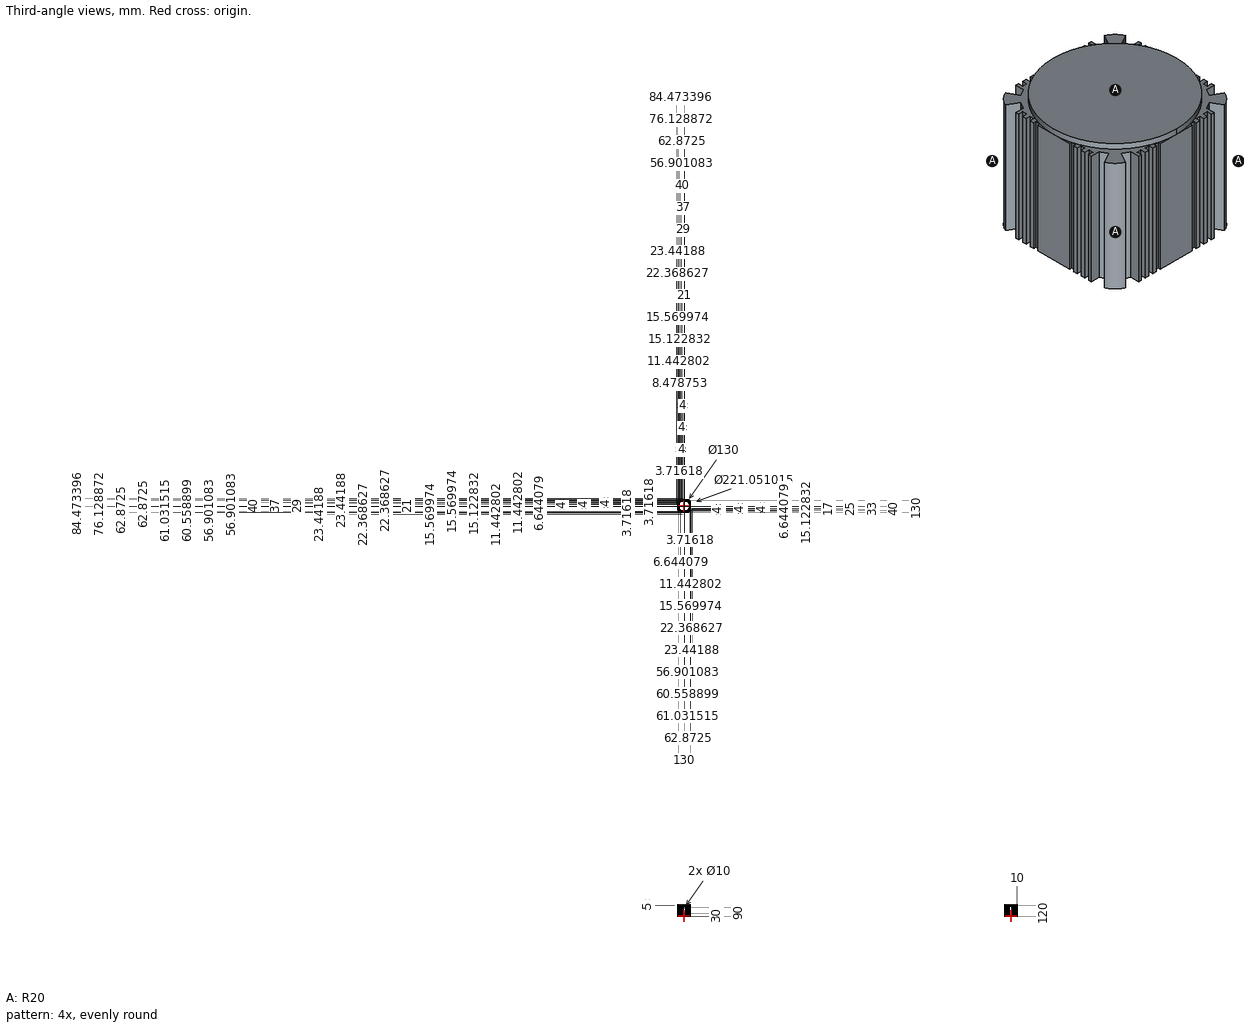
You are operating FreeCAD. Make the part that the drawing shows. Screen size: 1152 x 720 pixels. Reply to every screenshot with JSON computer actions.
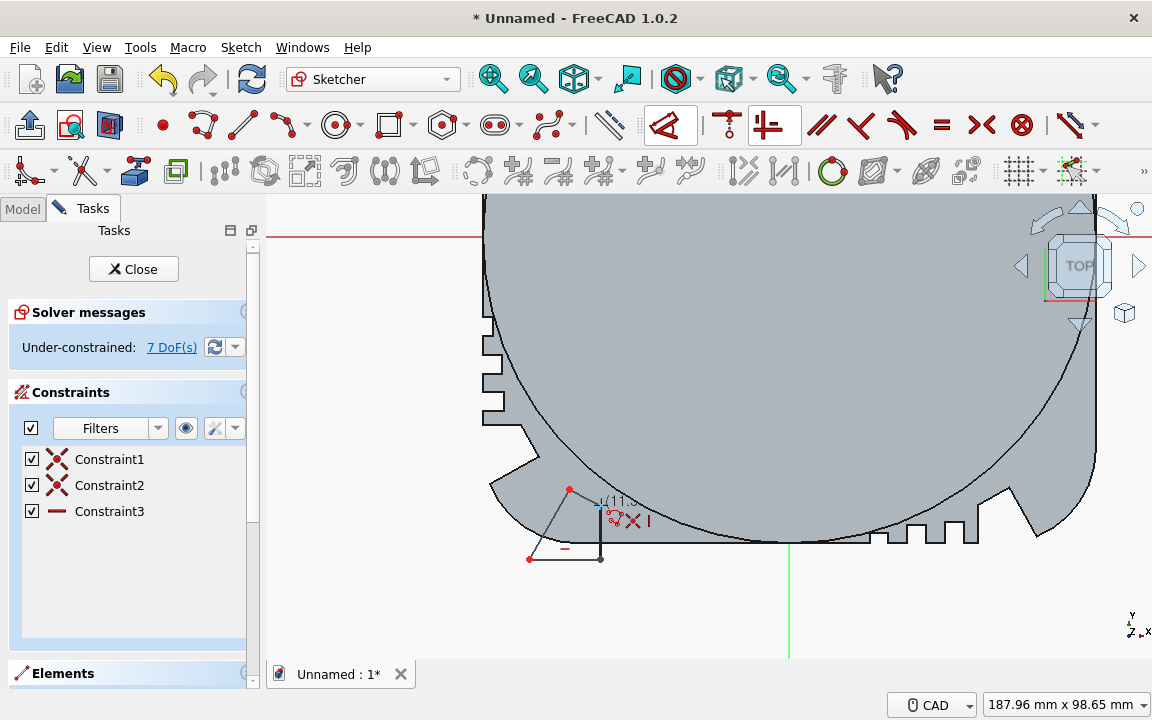
{"action": "left_click", "coordinate": [601, 506]}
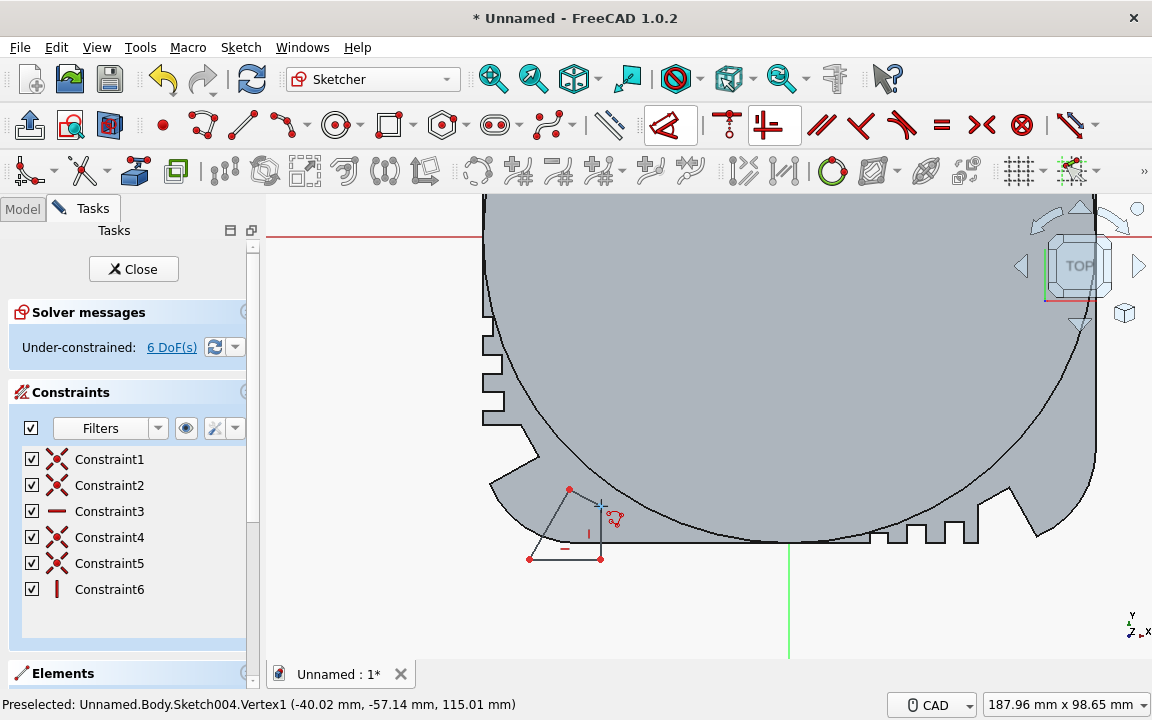
{"action": "left_click", "coordinate": [390, 126]}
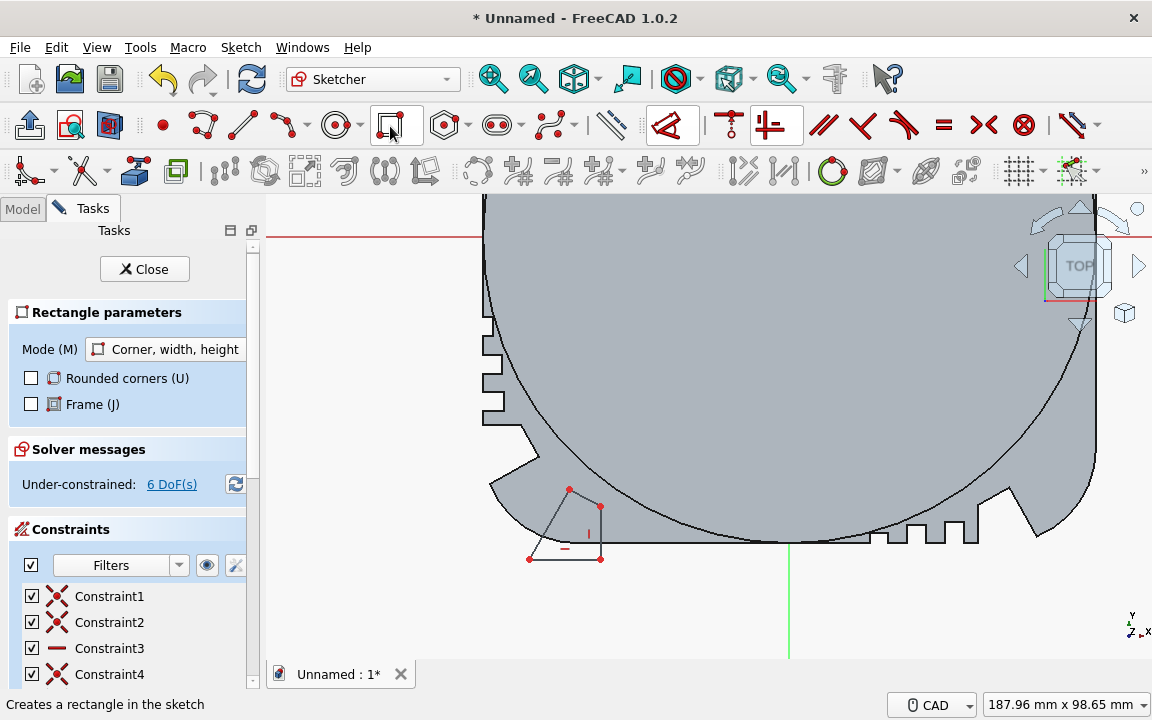
{"action": "left_click", "coordinate": [615, 522]}
{"action": "mouse_move", "coordinate": [634, 596]}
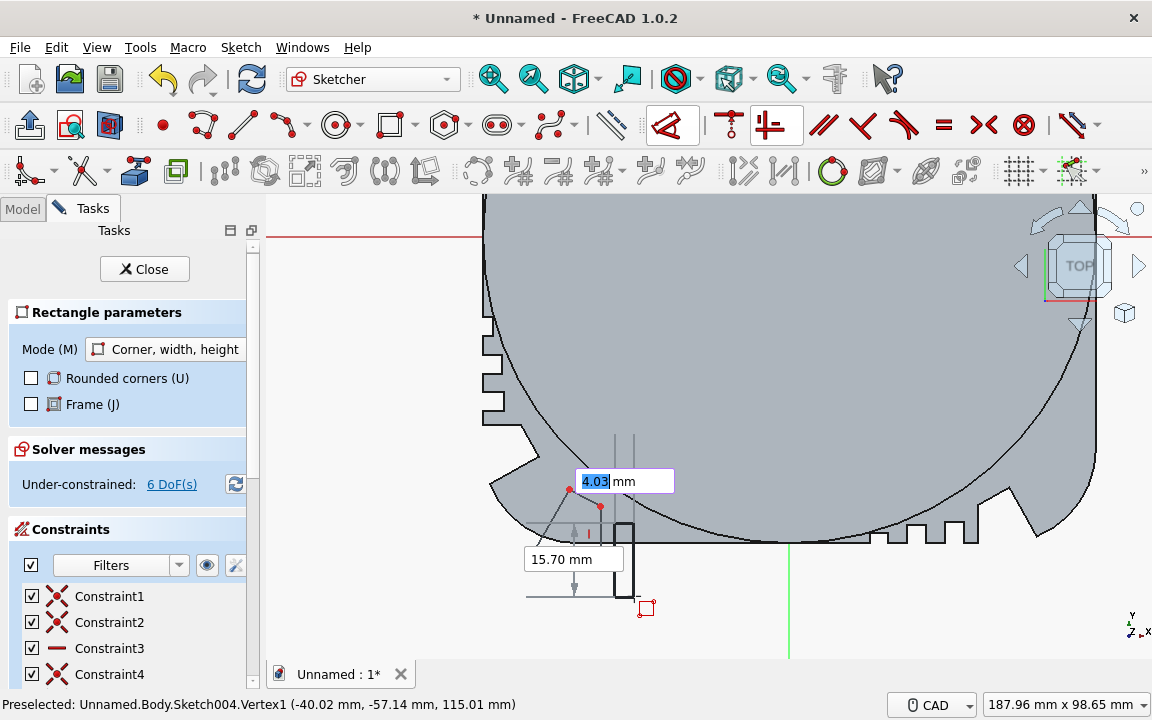
{"action": "type", "text": "4"}
{"action": "key", "text": "Tab"}
{"action": "type", "text": "15.569974"}
{"action": "key", "text": "Return"}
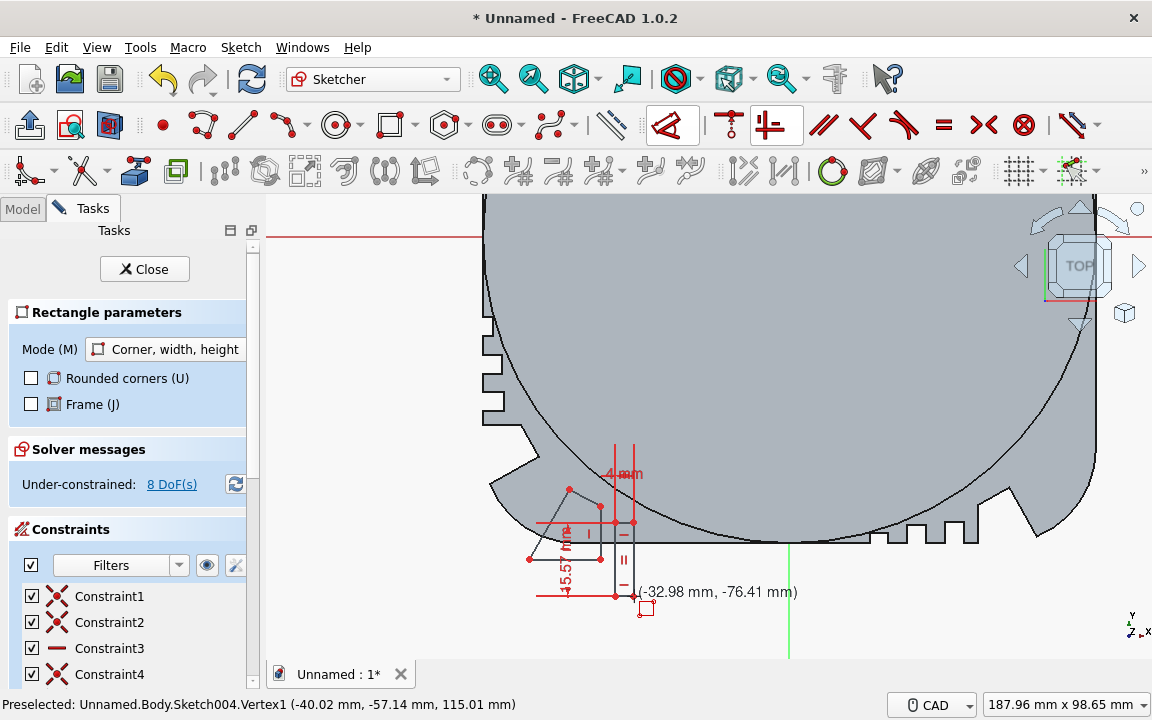
{"action": "left_click", "coordinate": [653, 525]}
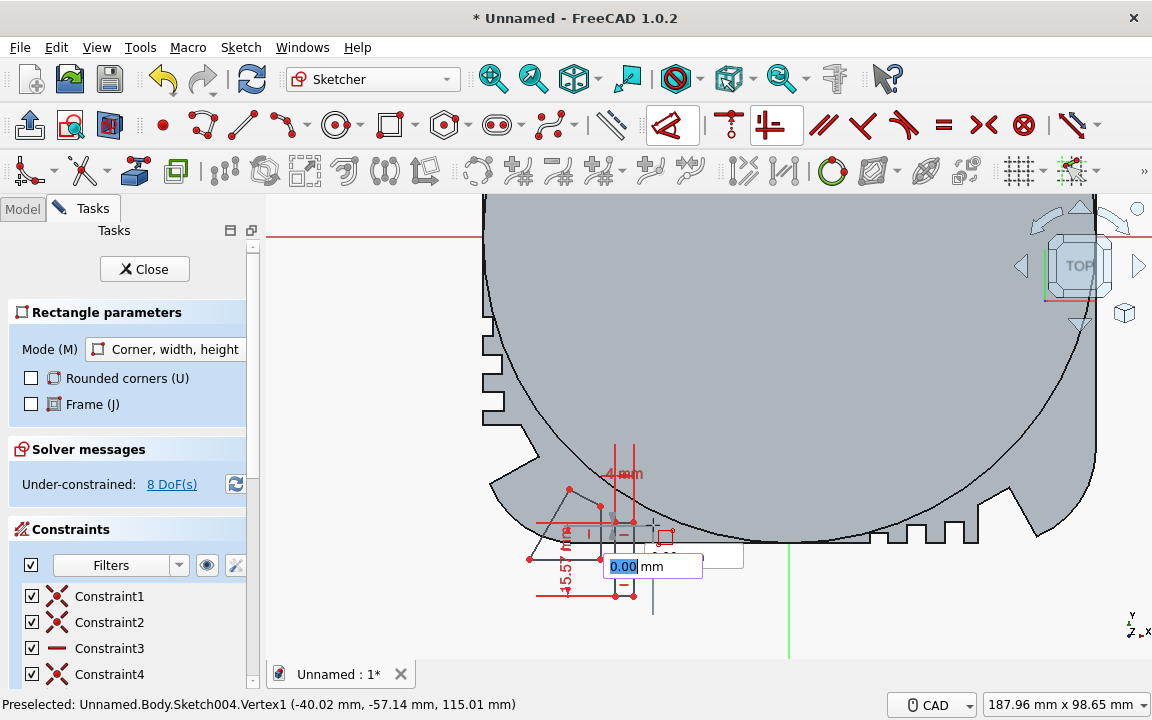
{"action": "scroll", "coordinate": [602, 404], "scroll_direction": "down", "scroll_amount": 2}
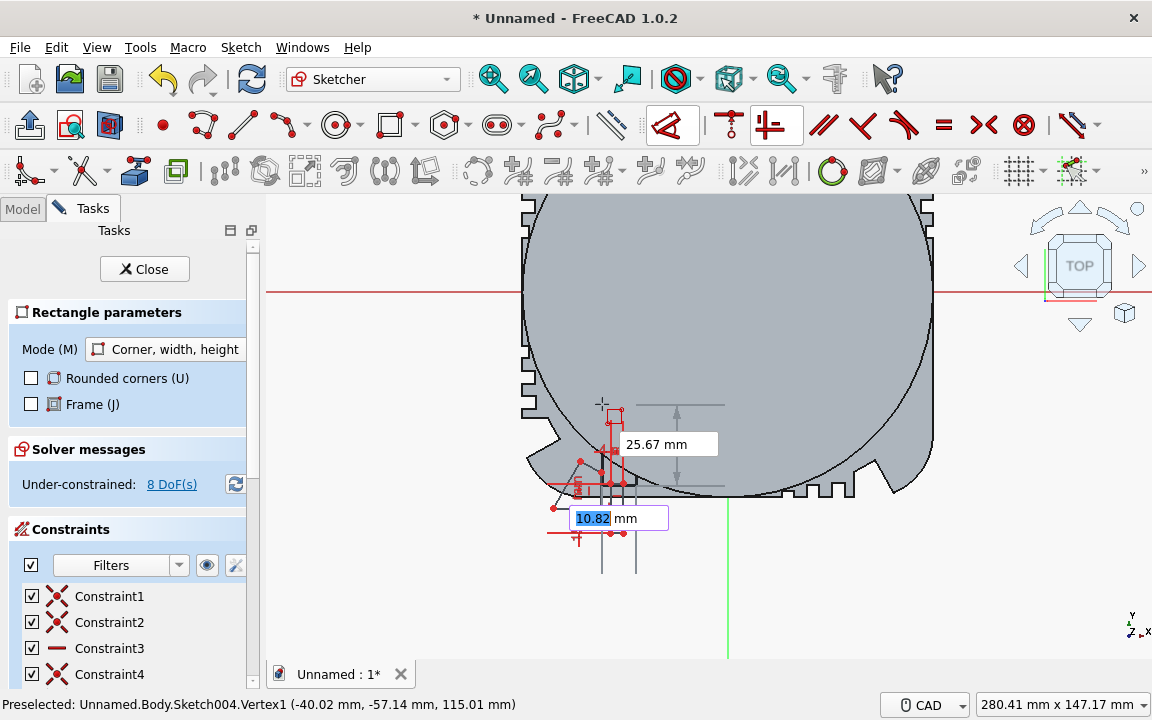
{"action": "left_click", "coordinate": [649, 559]}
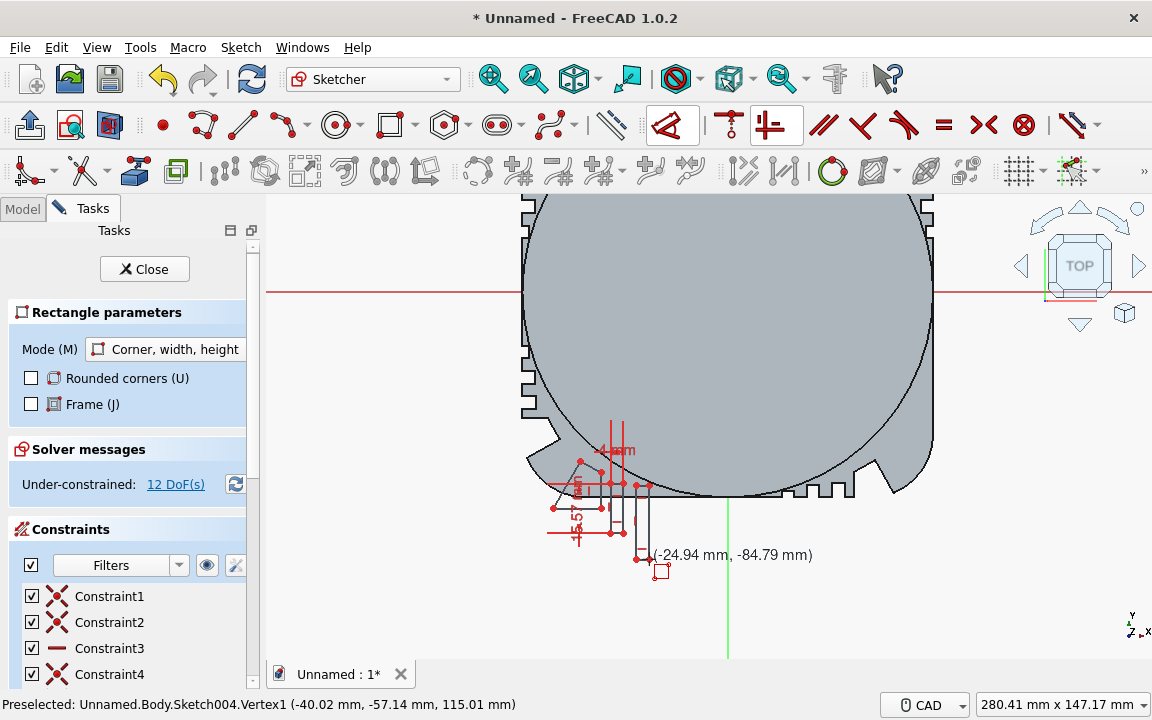
{"action": "scroll", "coordinate": [661, 491], "scroll_direction": "up", "scroll_amount": 2}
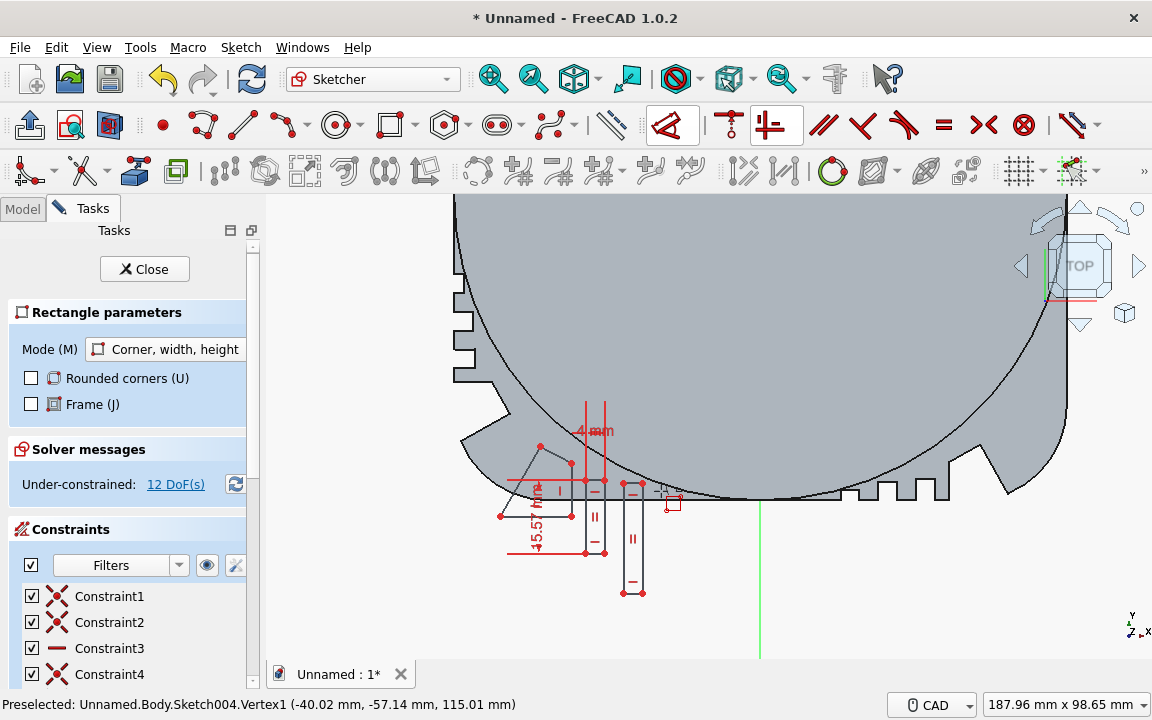
{"action": "left_click", "coordinate": [661, 490]}
{"action": "mouse_move", "coordinate": [680, 596]}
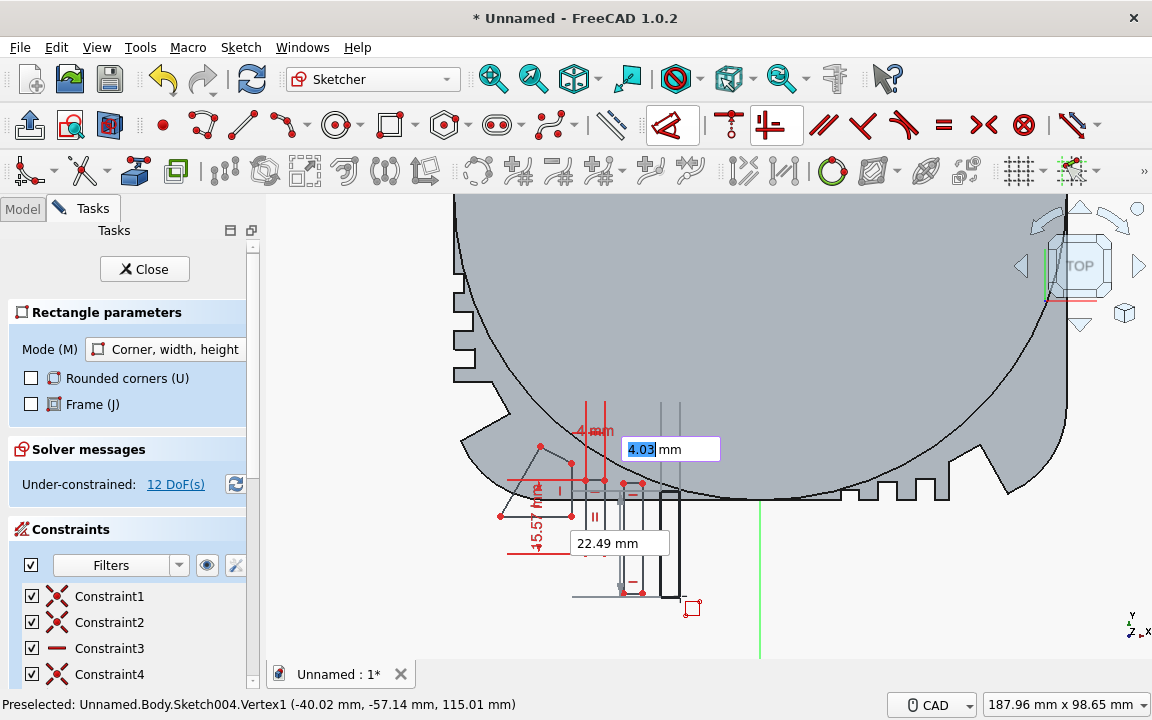
{"action": "type", "text": "4"}
{"action": "key", "text": "Tab"}
{"action": "type", "text": "22.368627"}
{"action": "key", "text": "Return"}
{"action": "key", "text": "Escape"}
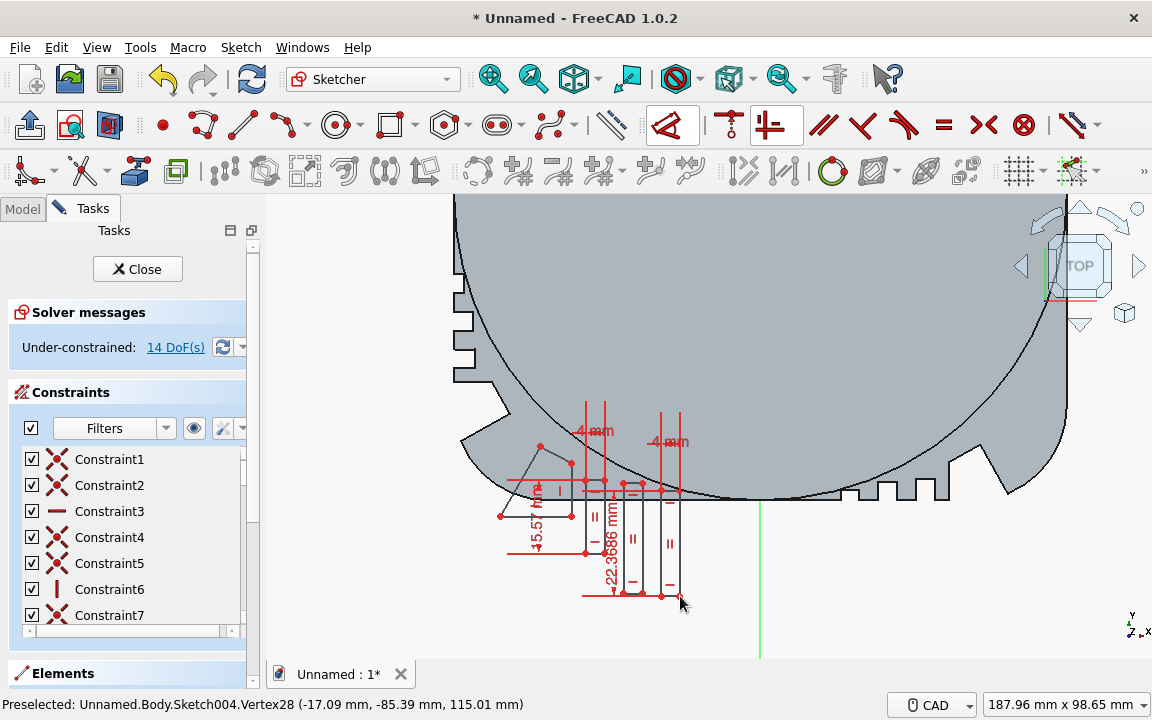
{"action": "scroll", "coordinate": [633, 594], "scroll_direction": "up", "scroll_amount": 4}